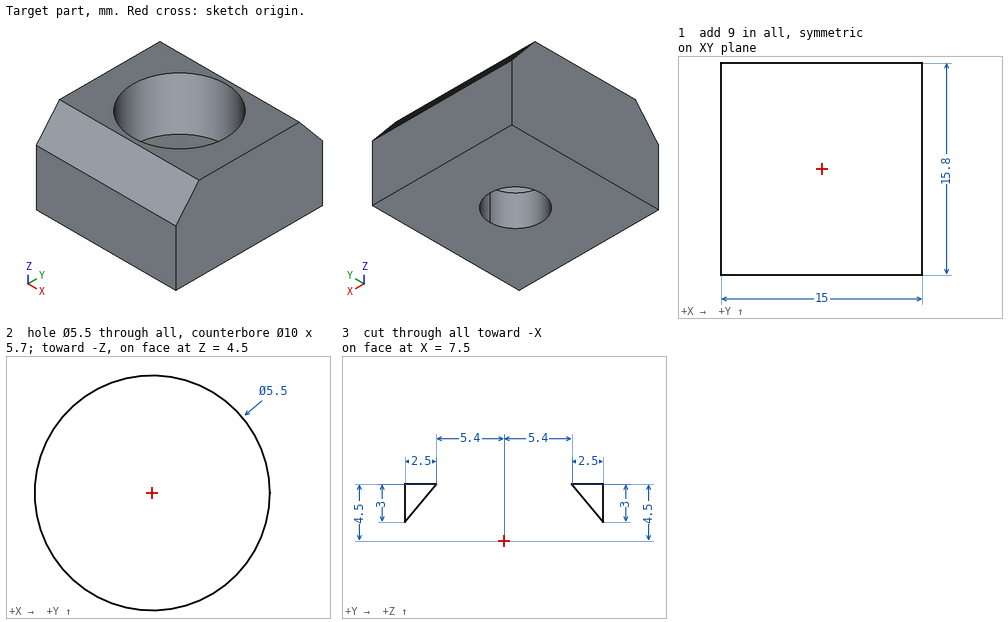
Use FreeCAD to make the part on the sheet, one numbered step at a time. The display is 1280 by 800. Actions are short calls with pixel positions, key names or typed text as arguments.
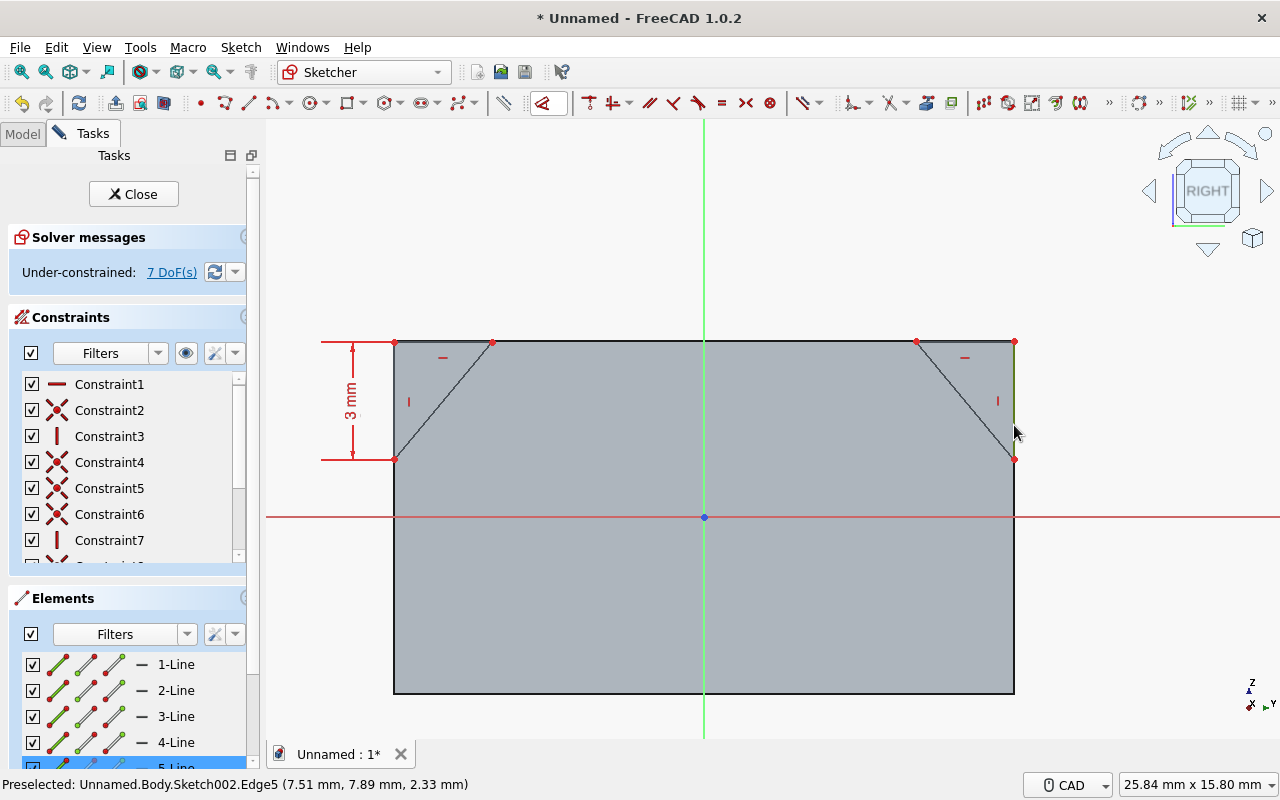
key(i)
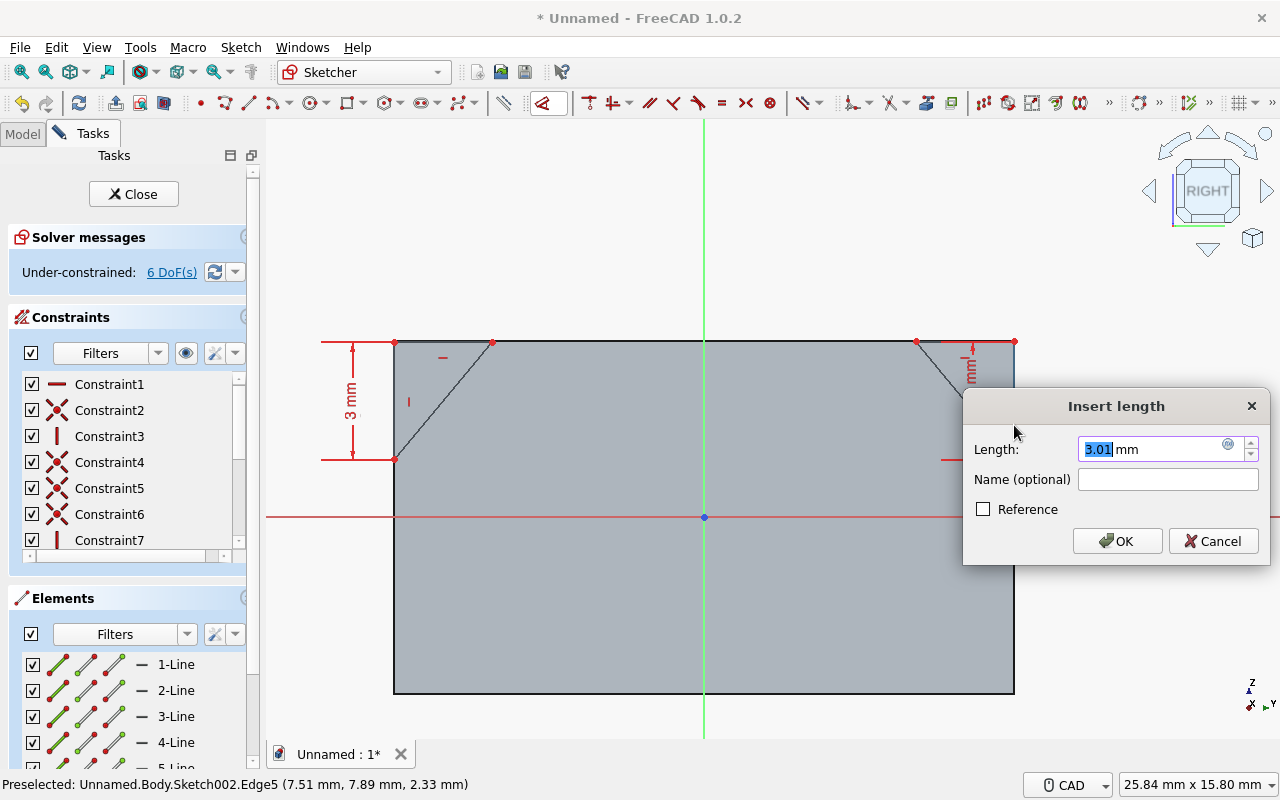
text(3)
key(Return)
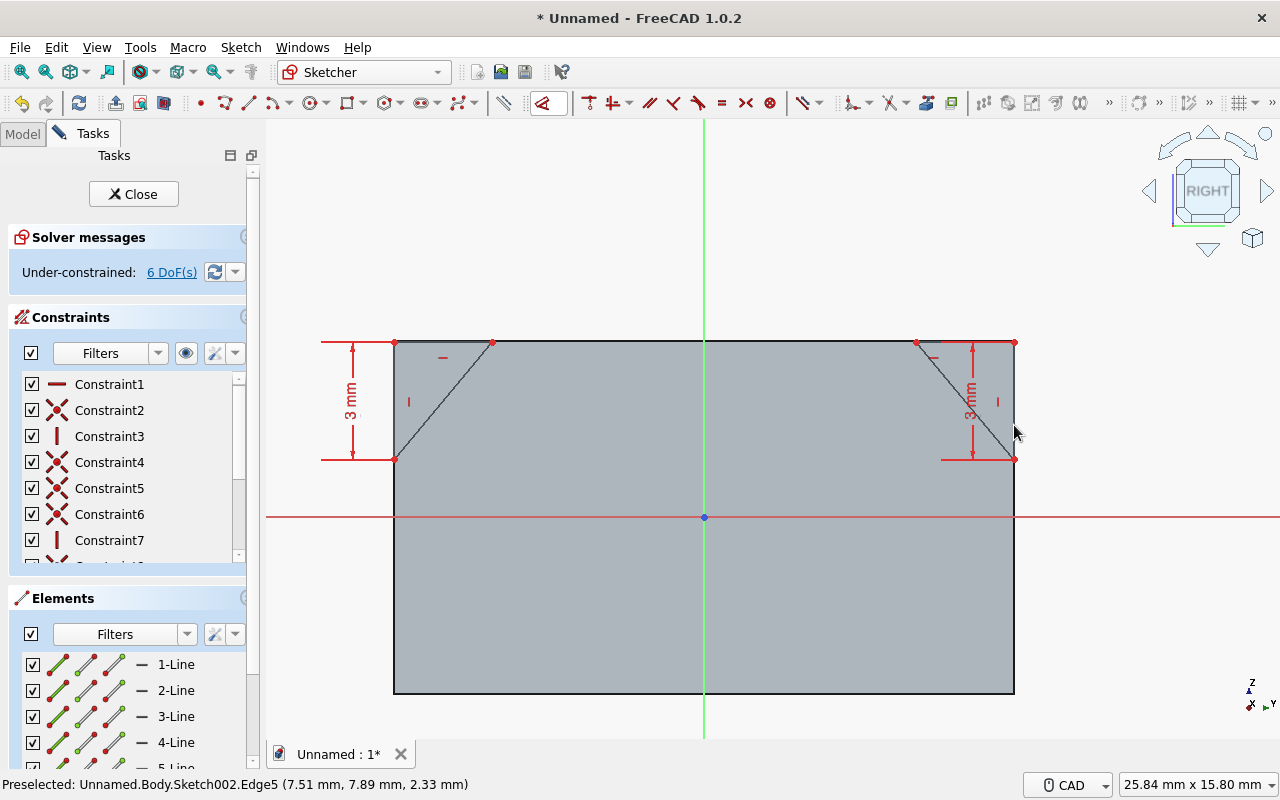
click(463, 342)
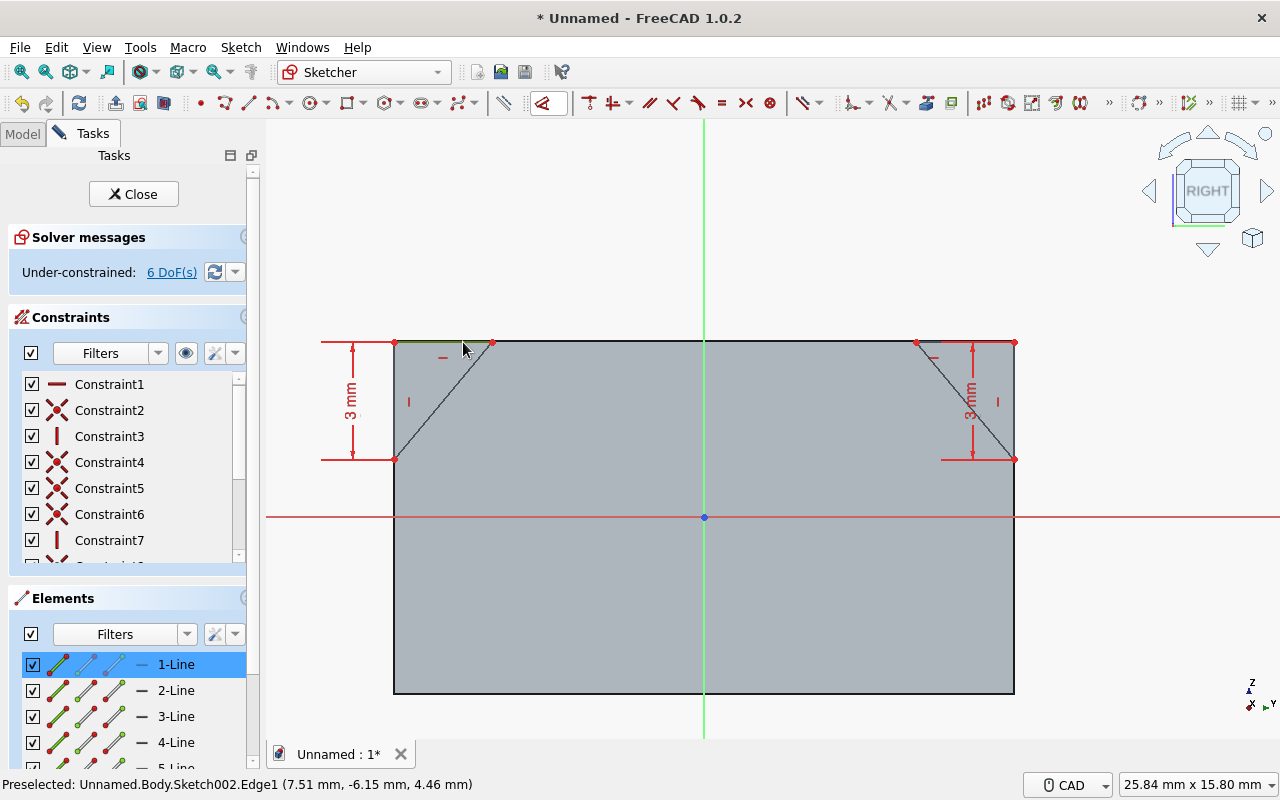
key(l)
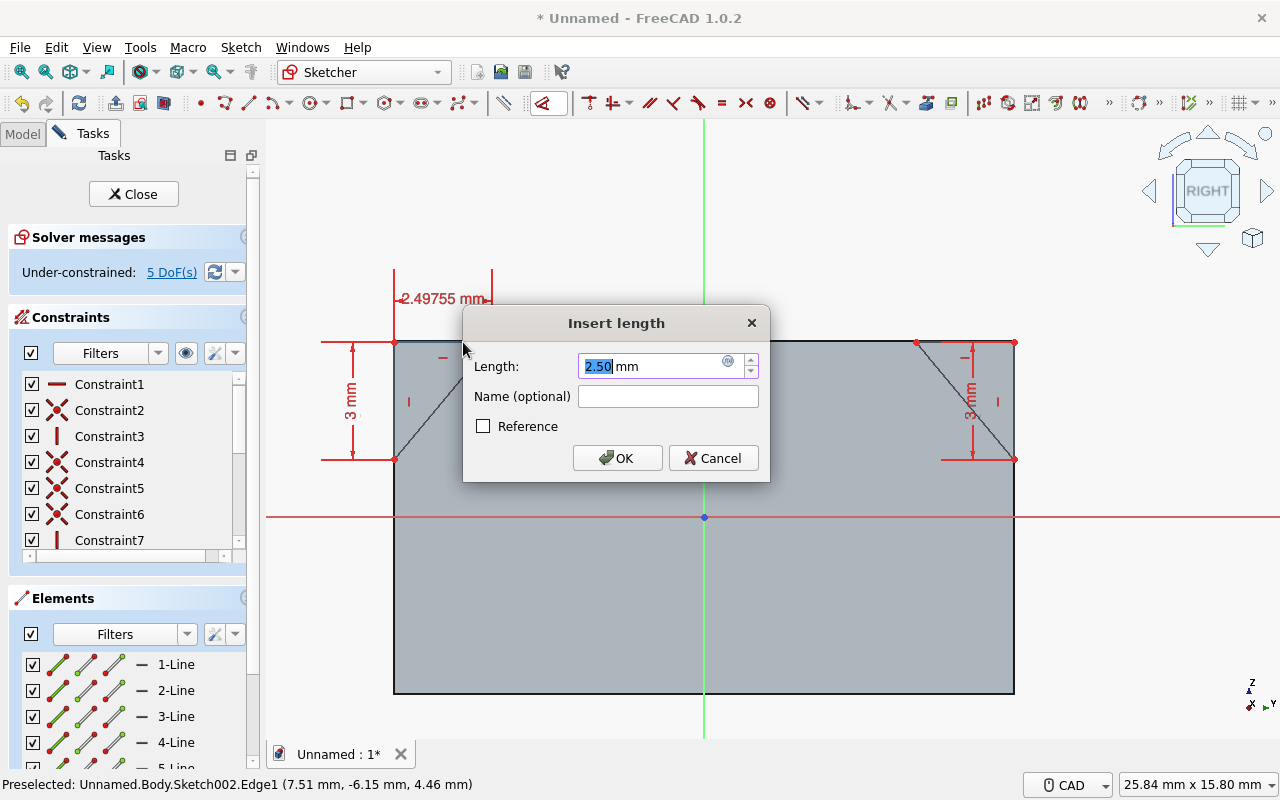
text(2.5)
key(Return)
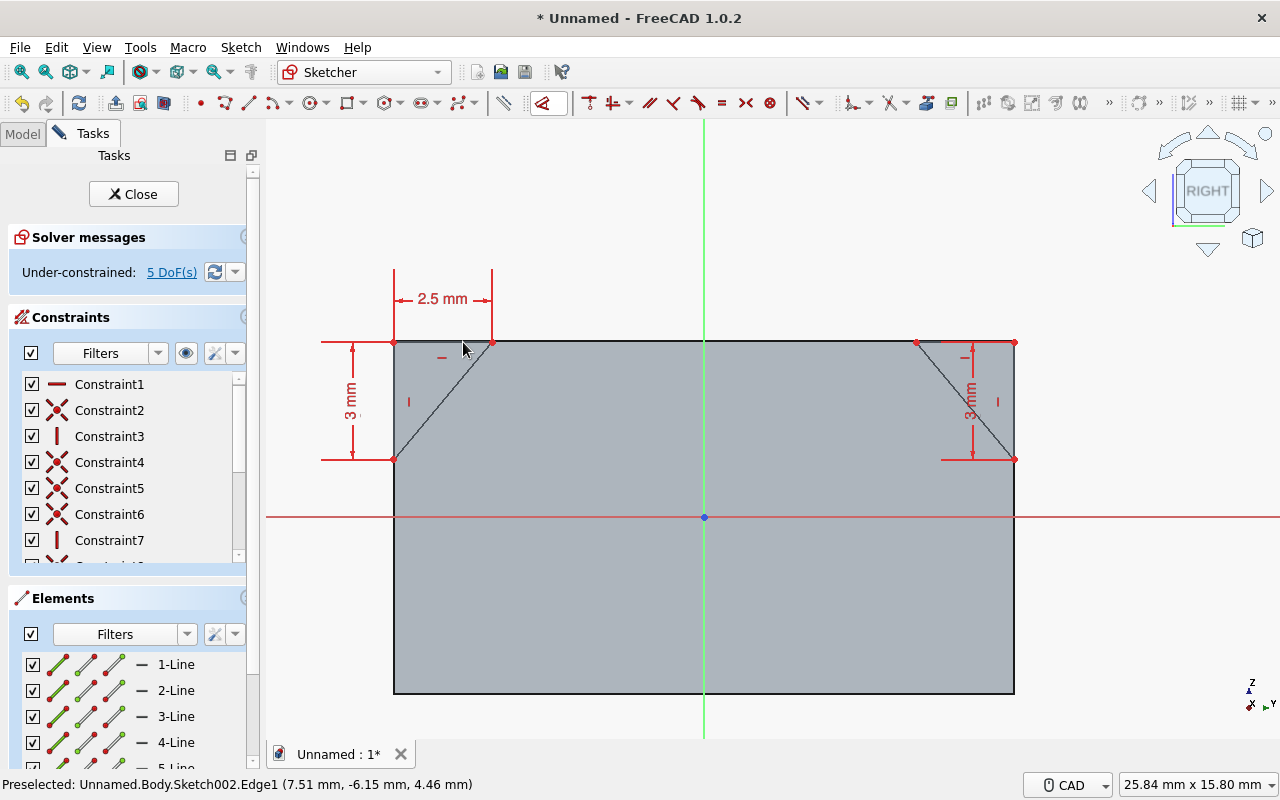
click(985, 342)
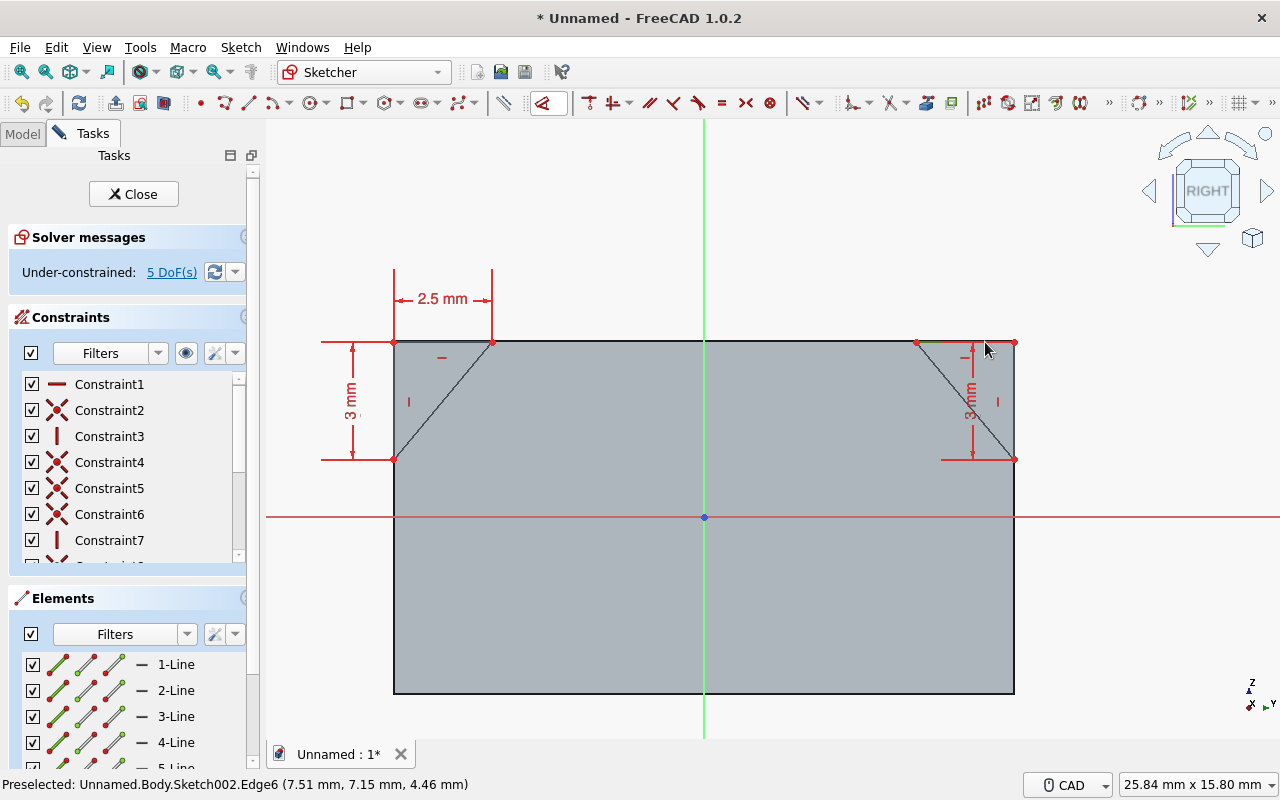
click(562, 104)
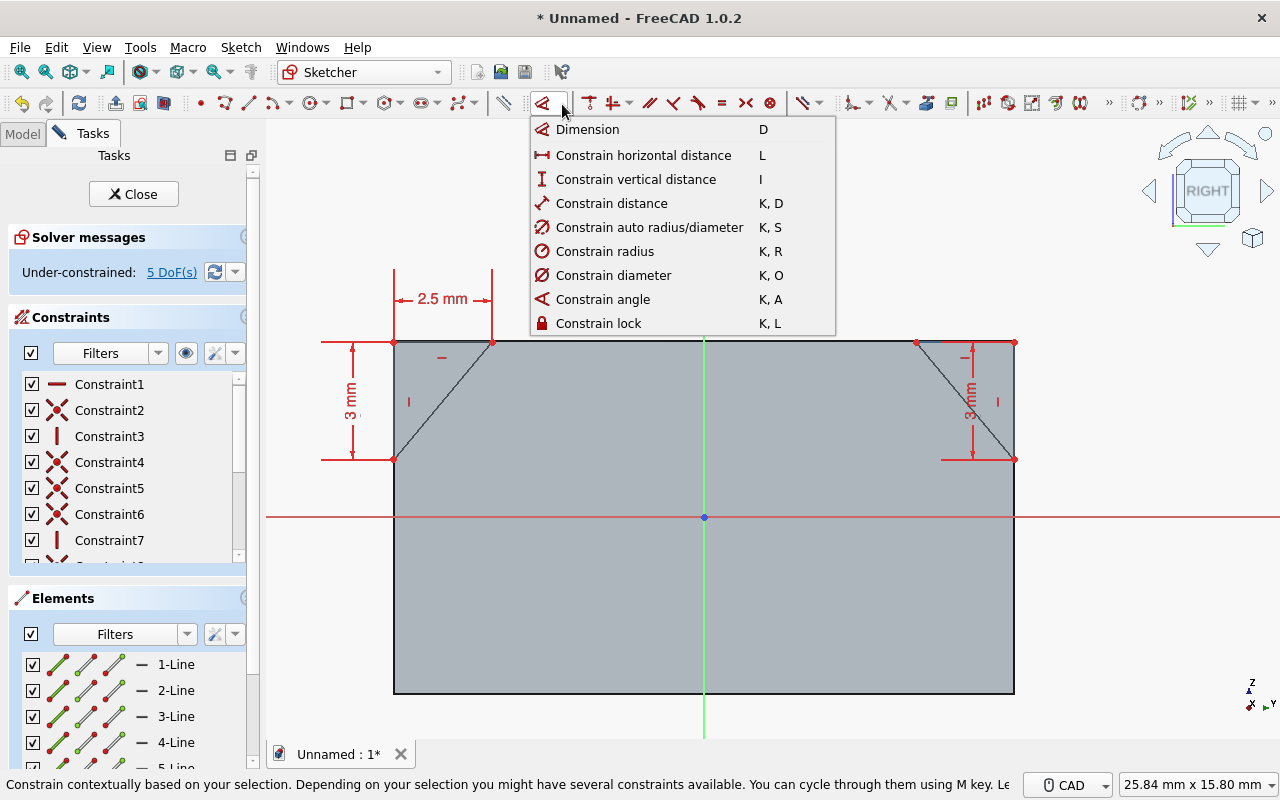
click(683, 155)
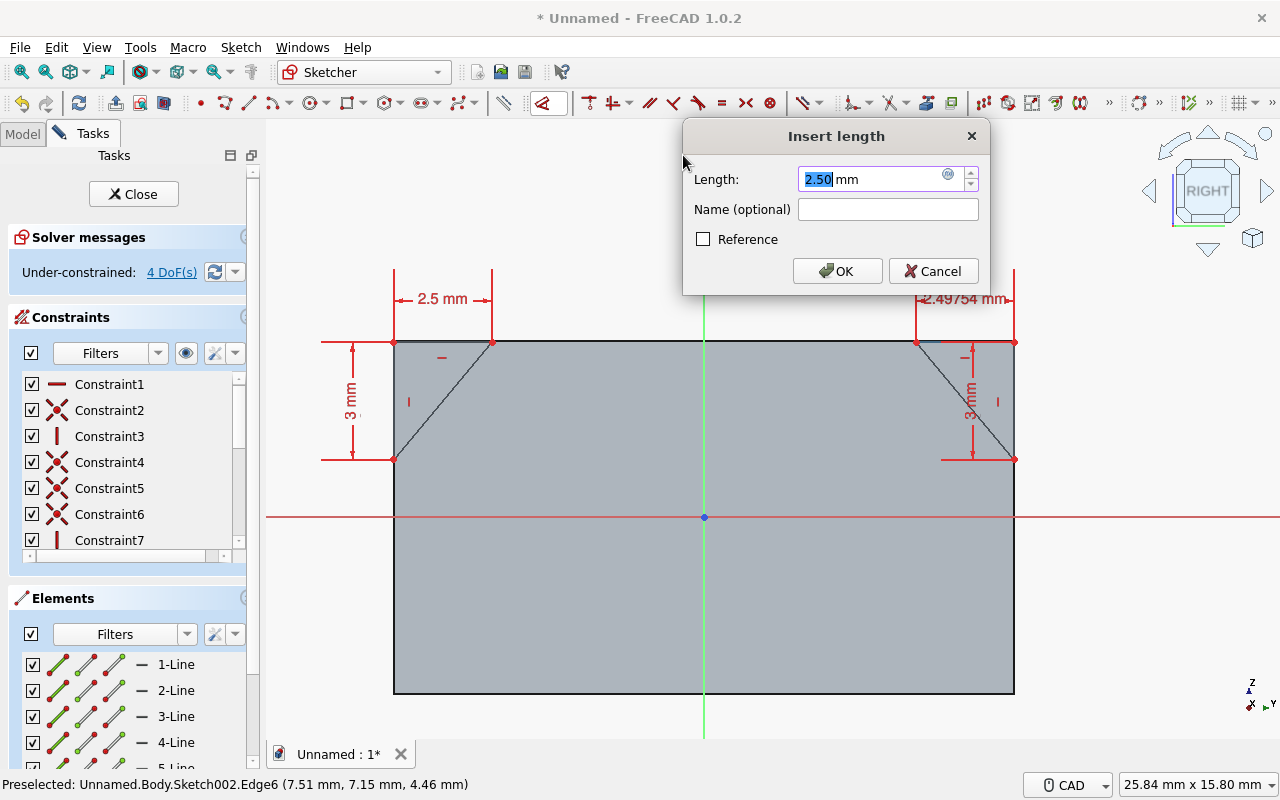
text(2.5)
key(Return)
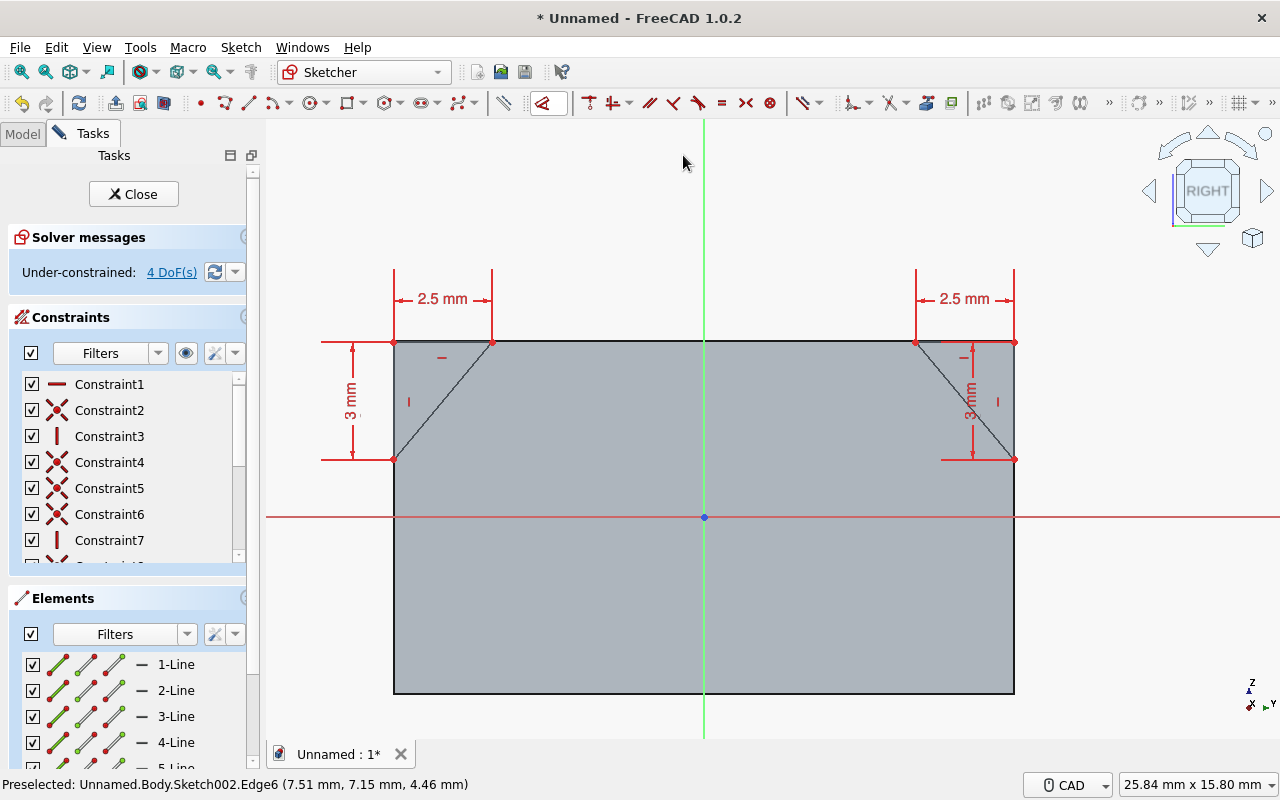
click(492, 342)